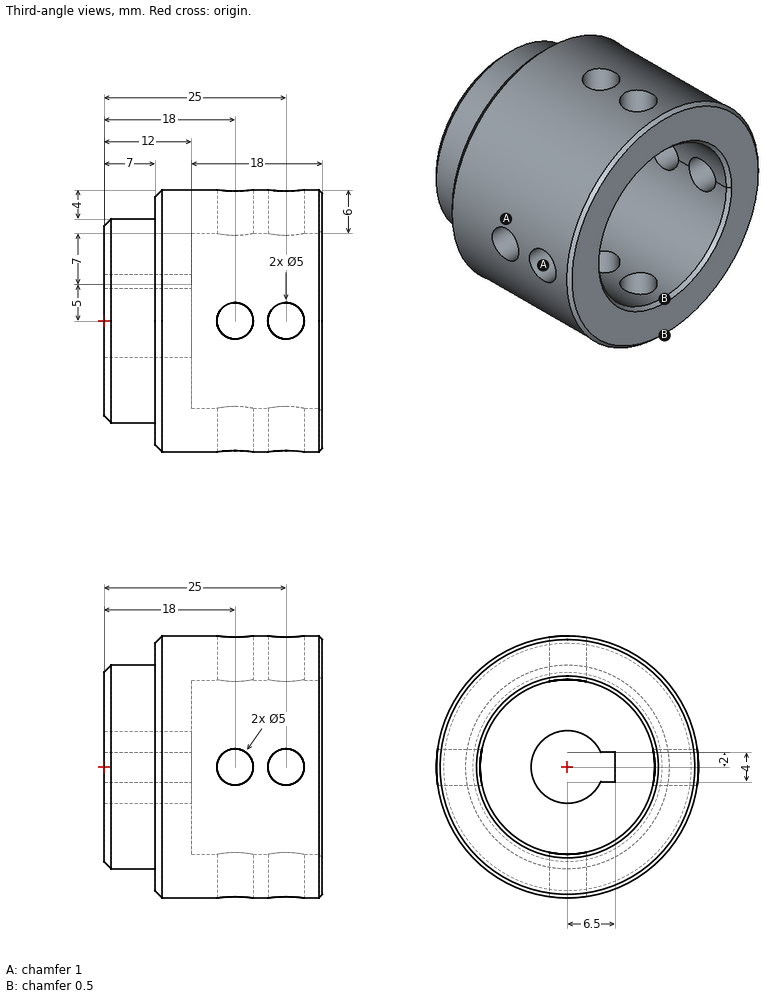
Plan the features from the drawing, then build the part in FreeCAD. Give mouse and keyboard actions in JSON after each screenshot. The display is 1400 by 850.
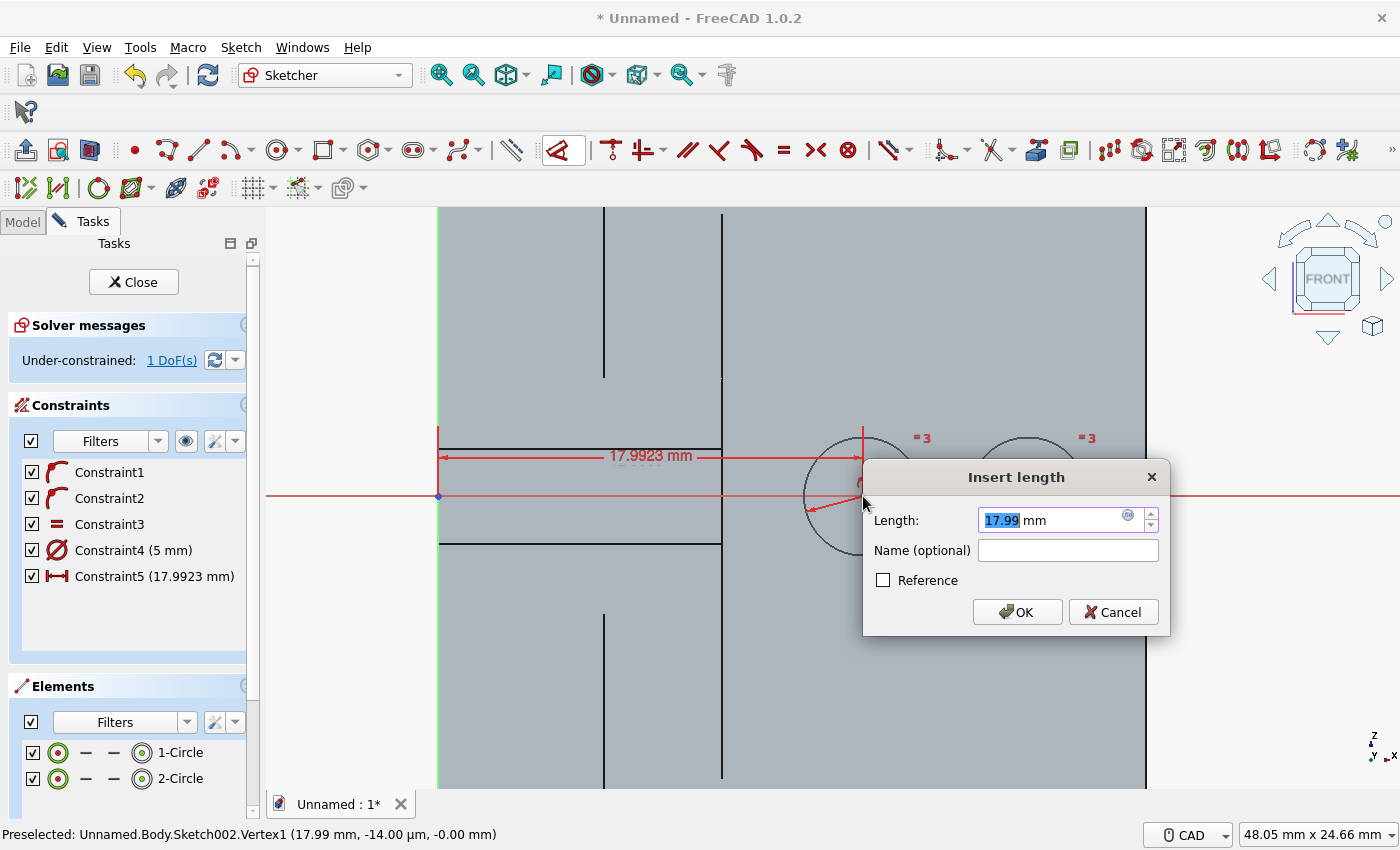
{"action": "type", "text": "18"}
{"action": "key", "text": "Return"}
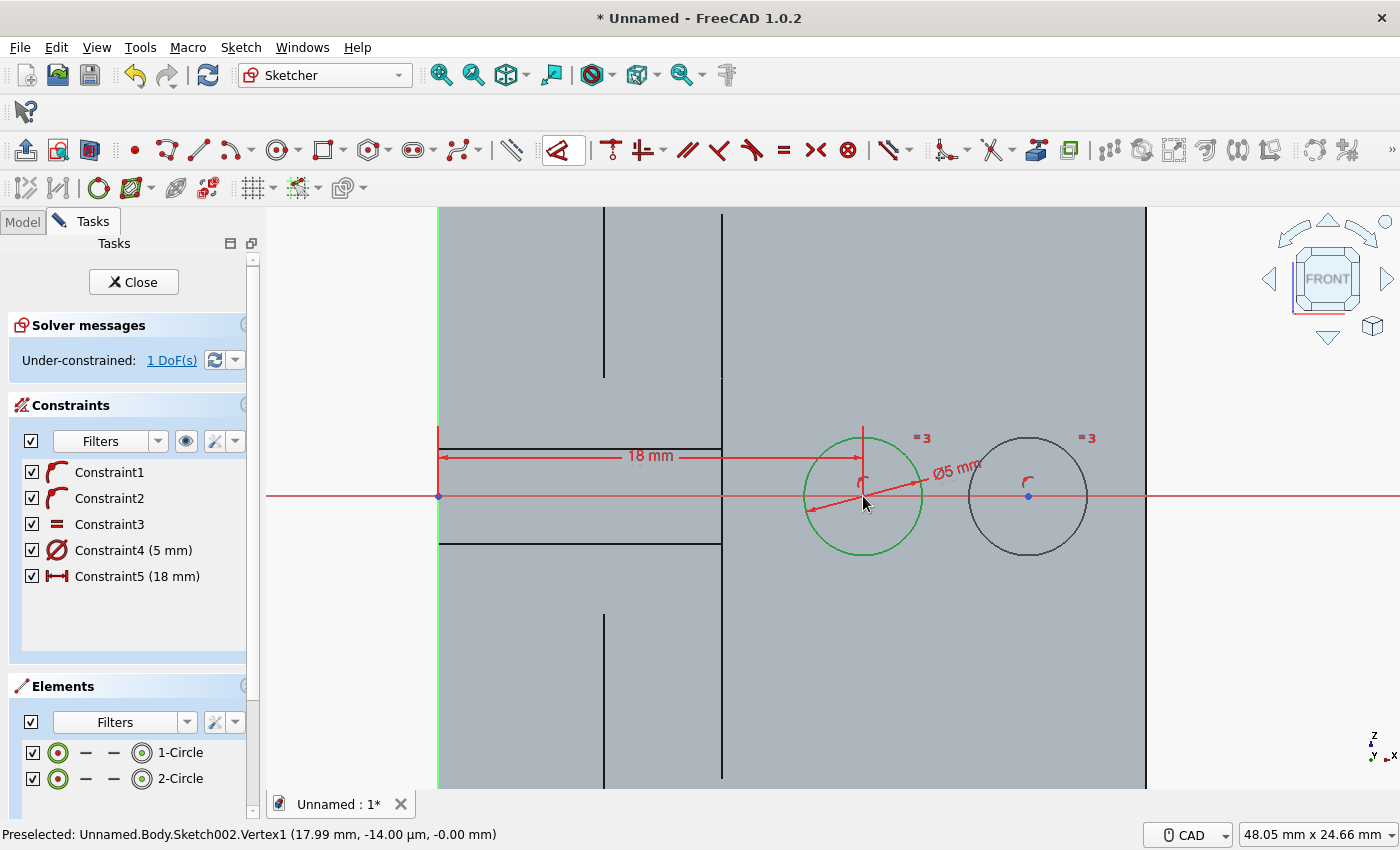
{"action": "left_click", "coordinate": [1028, 496]}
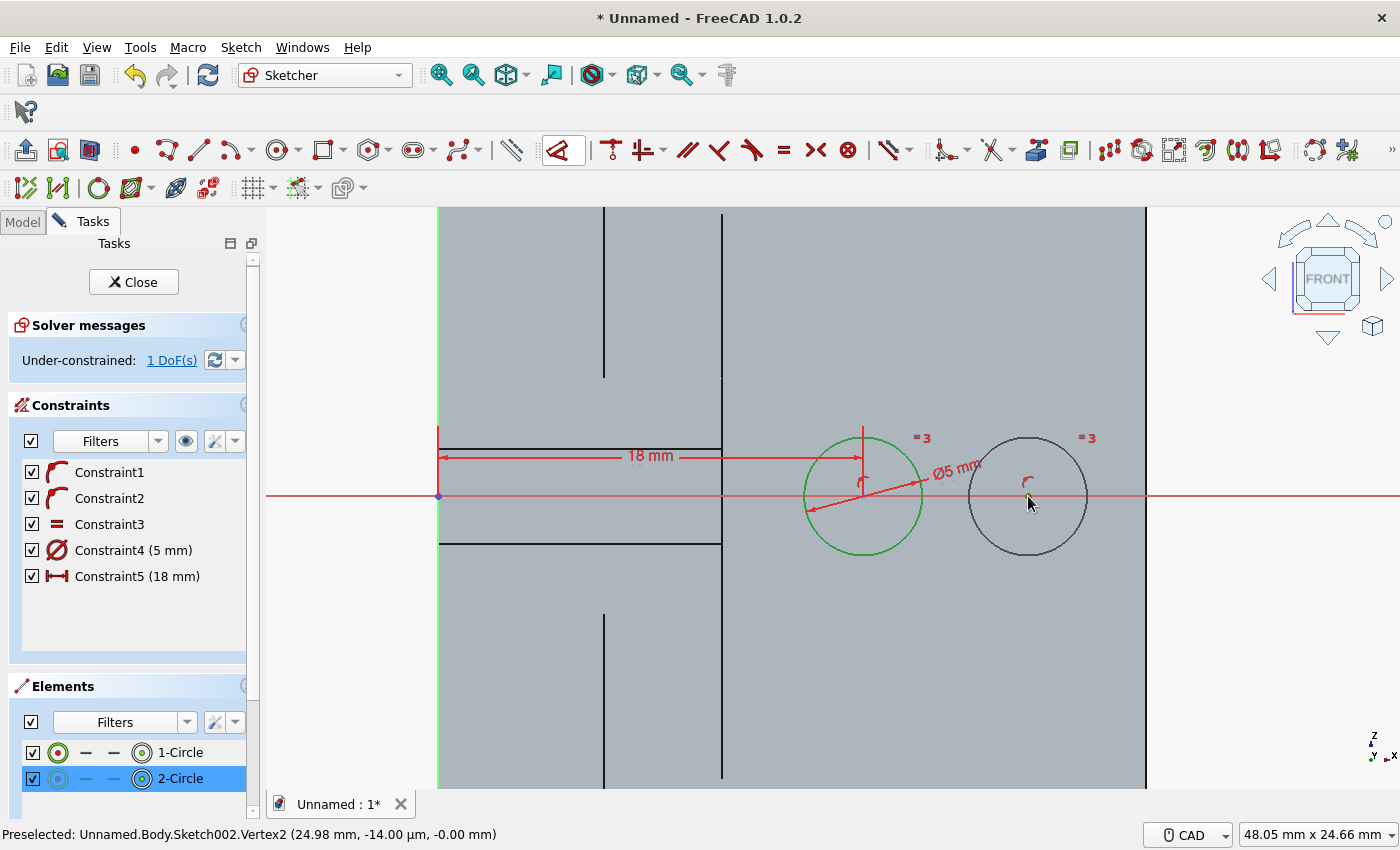
{"action": "left_click", "coordinate": [580, 150]}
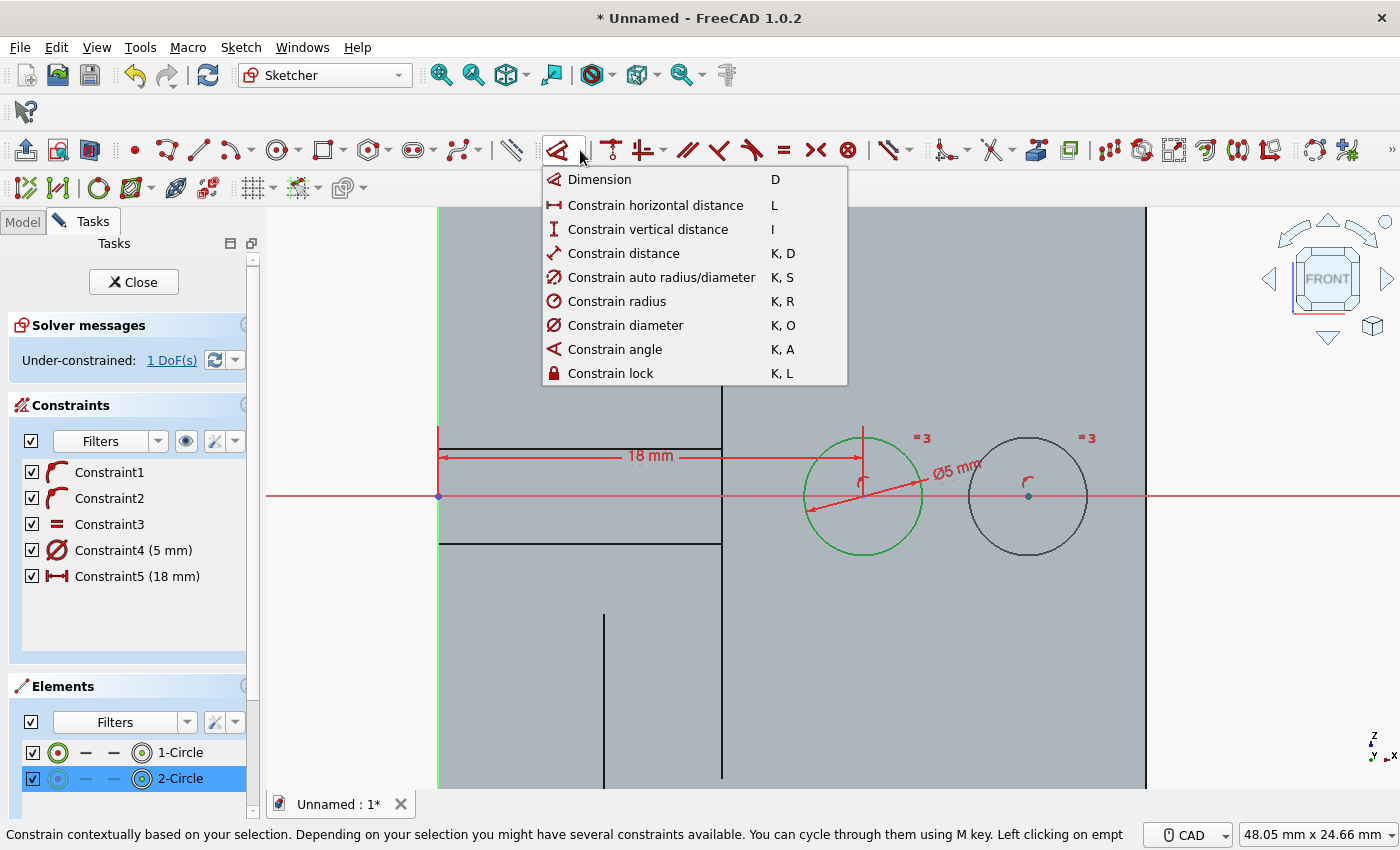
{"action": "left_click", "coordinate": [695, 205]}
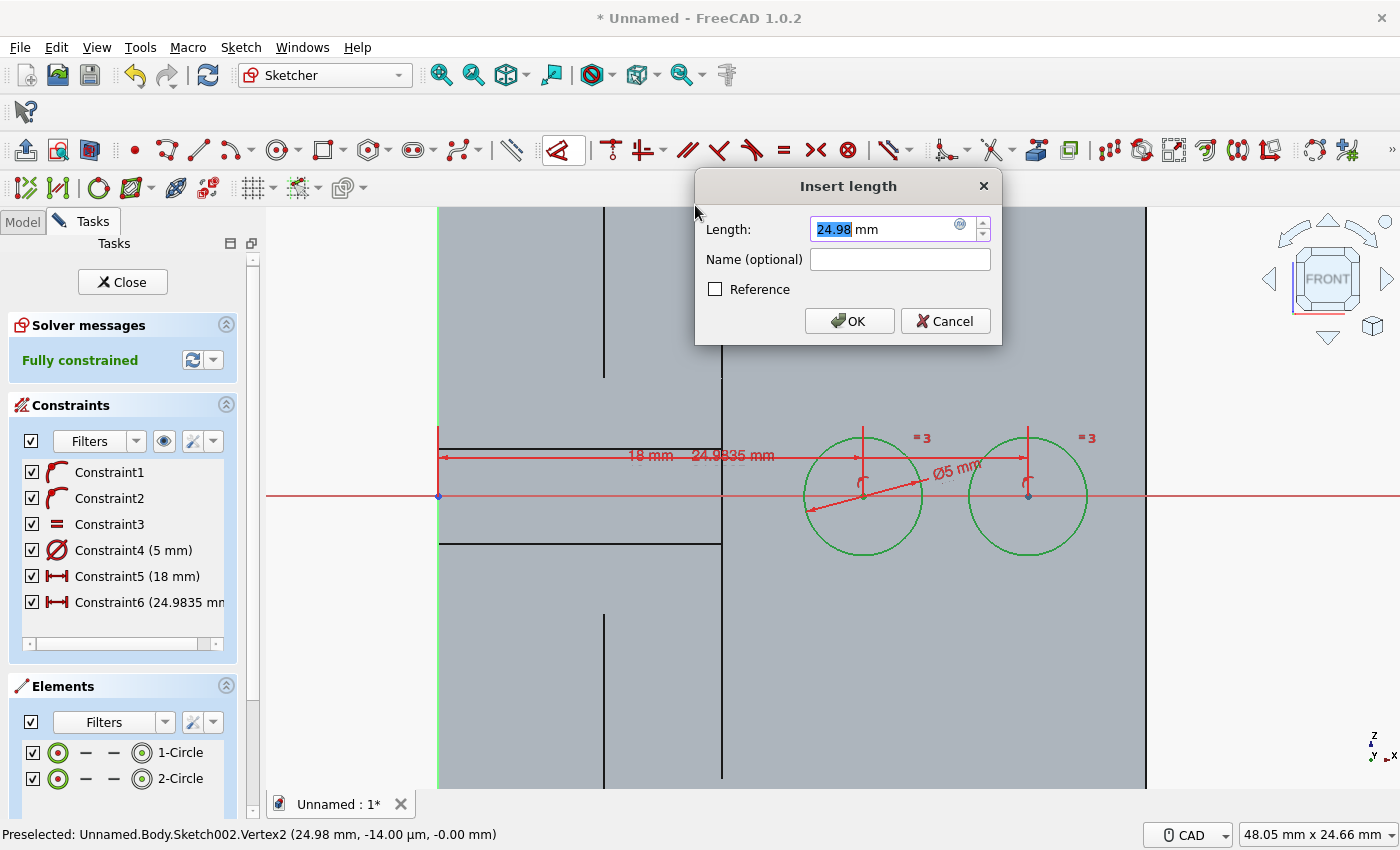
{"action": "type", "text": "25"}
{"action": "key", "text": "Return"}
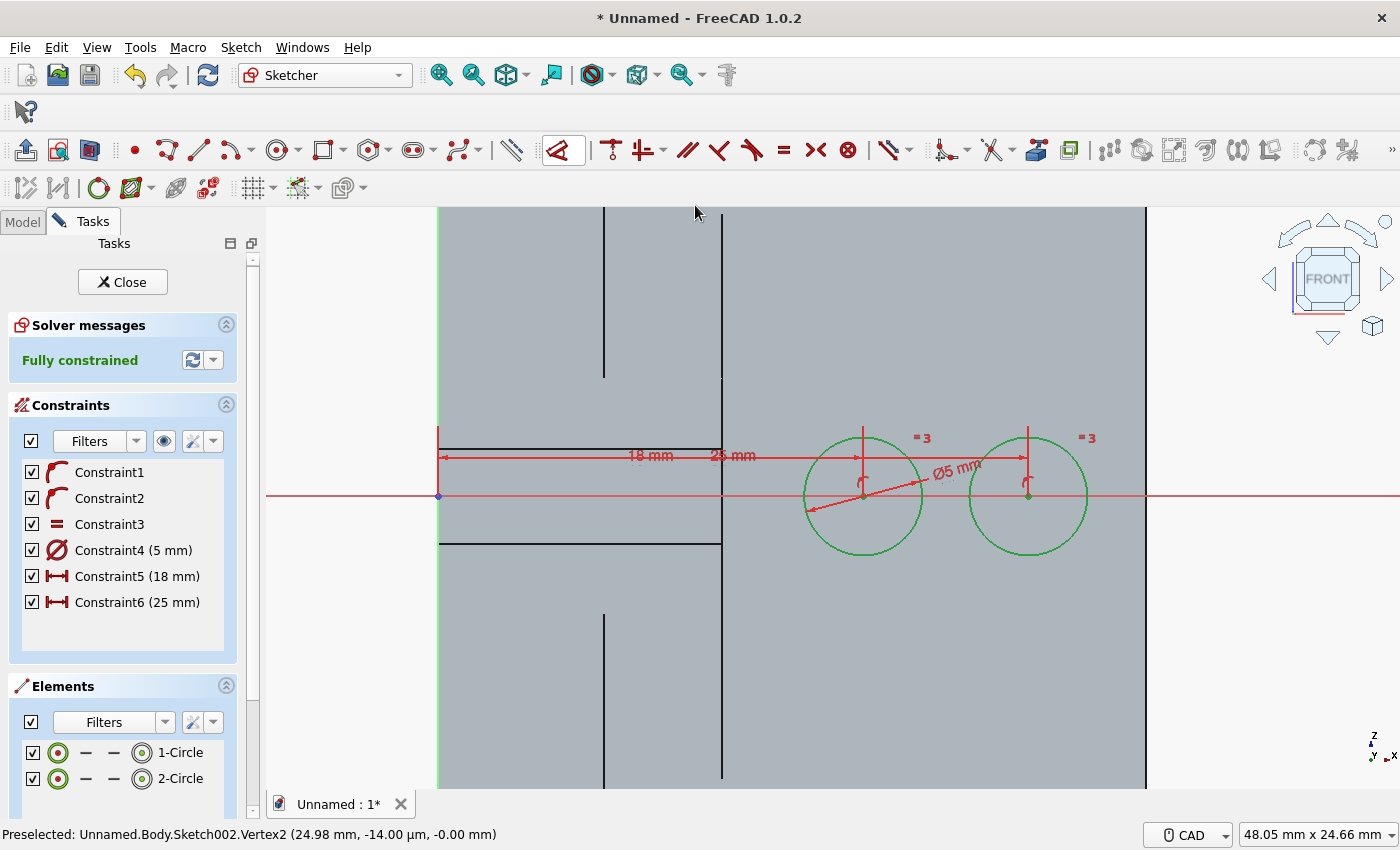
{"action": "left_click", "coordinate": [123, 282]}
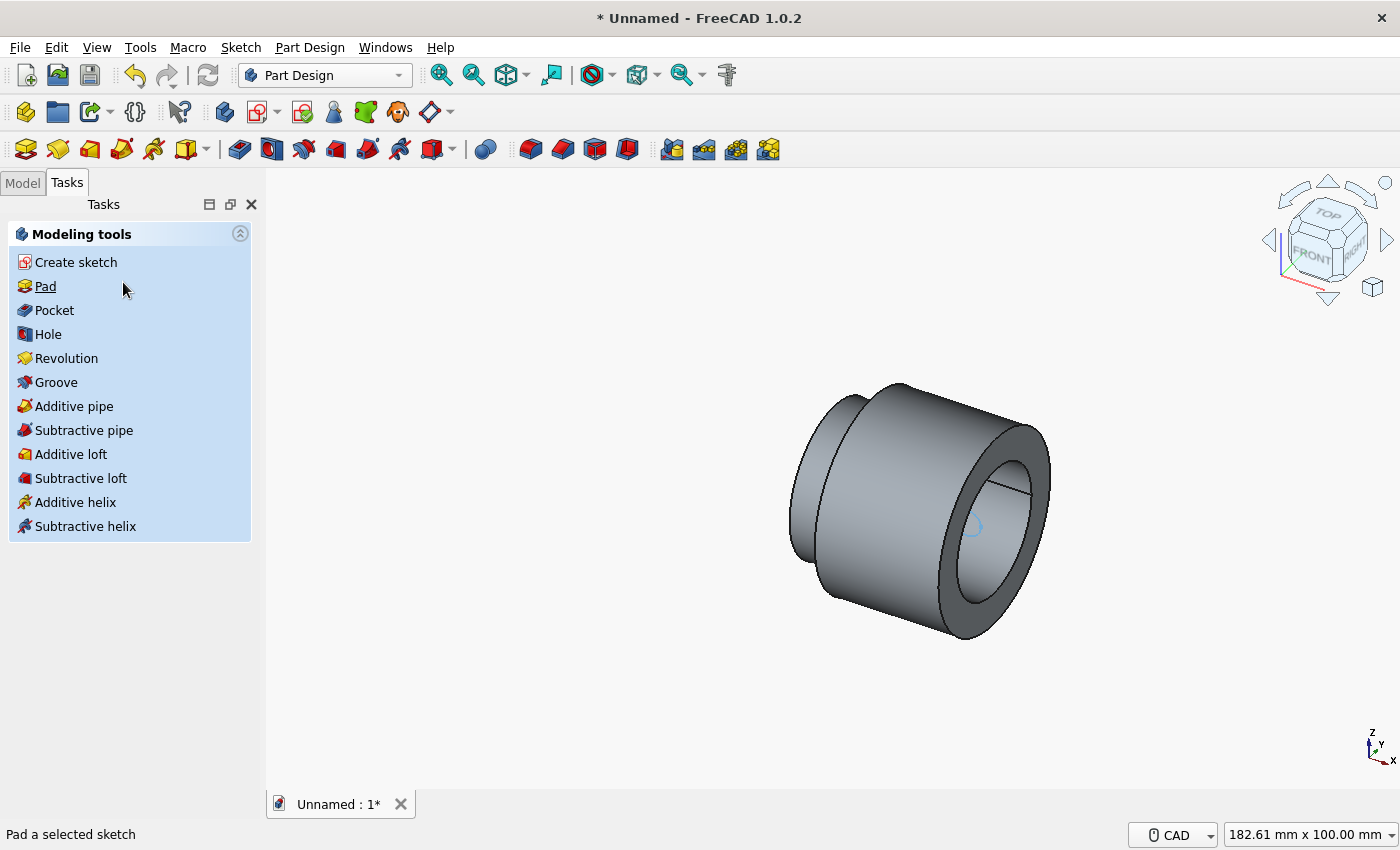
{"action": "left_click", "coordinate": [240, 150]}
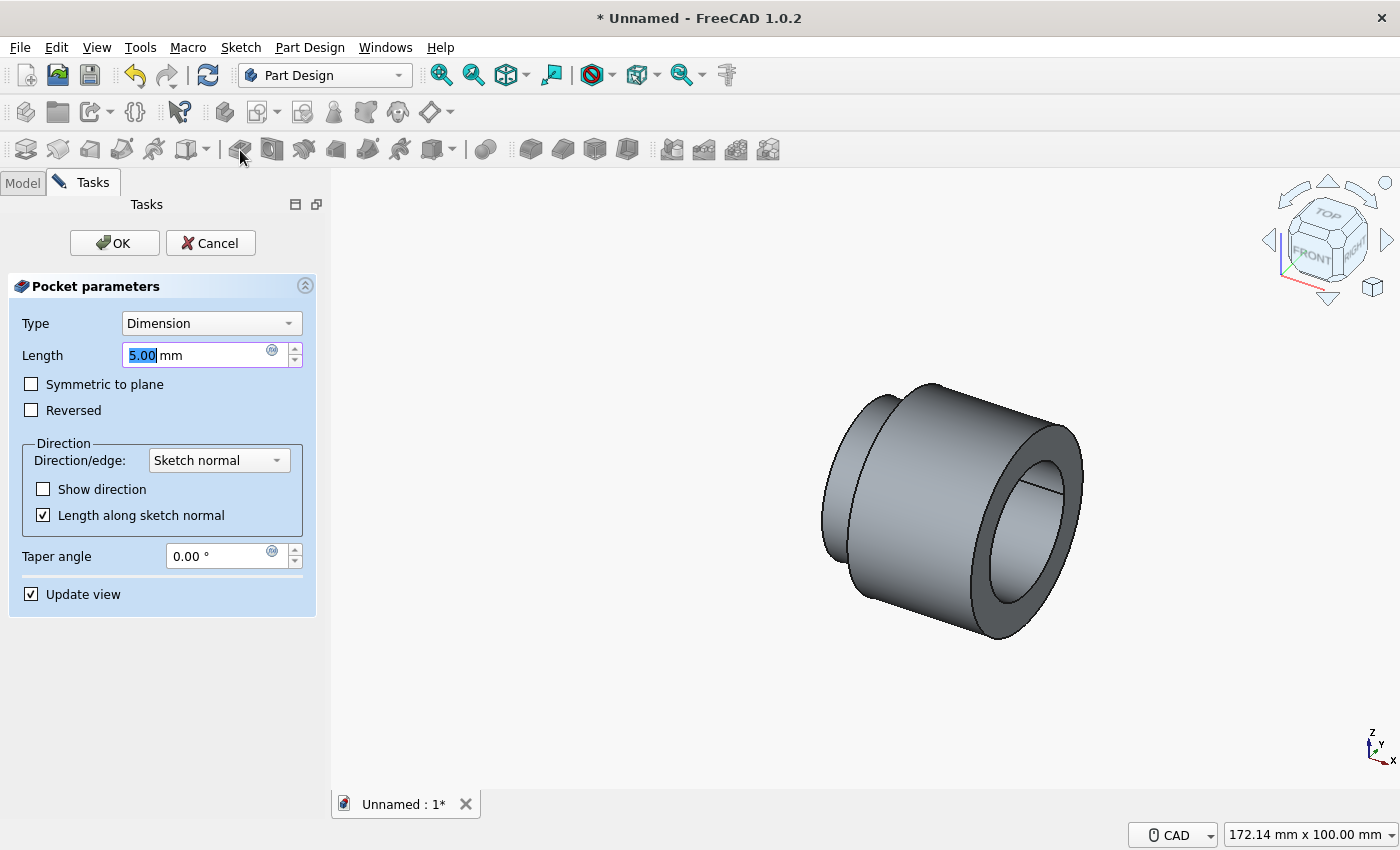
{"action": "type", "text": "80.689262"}
{"action": "key", "text": "Tab"}